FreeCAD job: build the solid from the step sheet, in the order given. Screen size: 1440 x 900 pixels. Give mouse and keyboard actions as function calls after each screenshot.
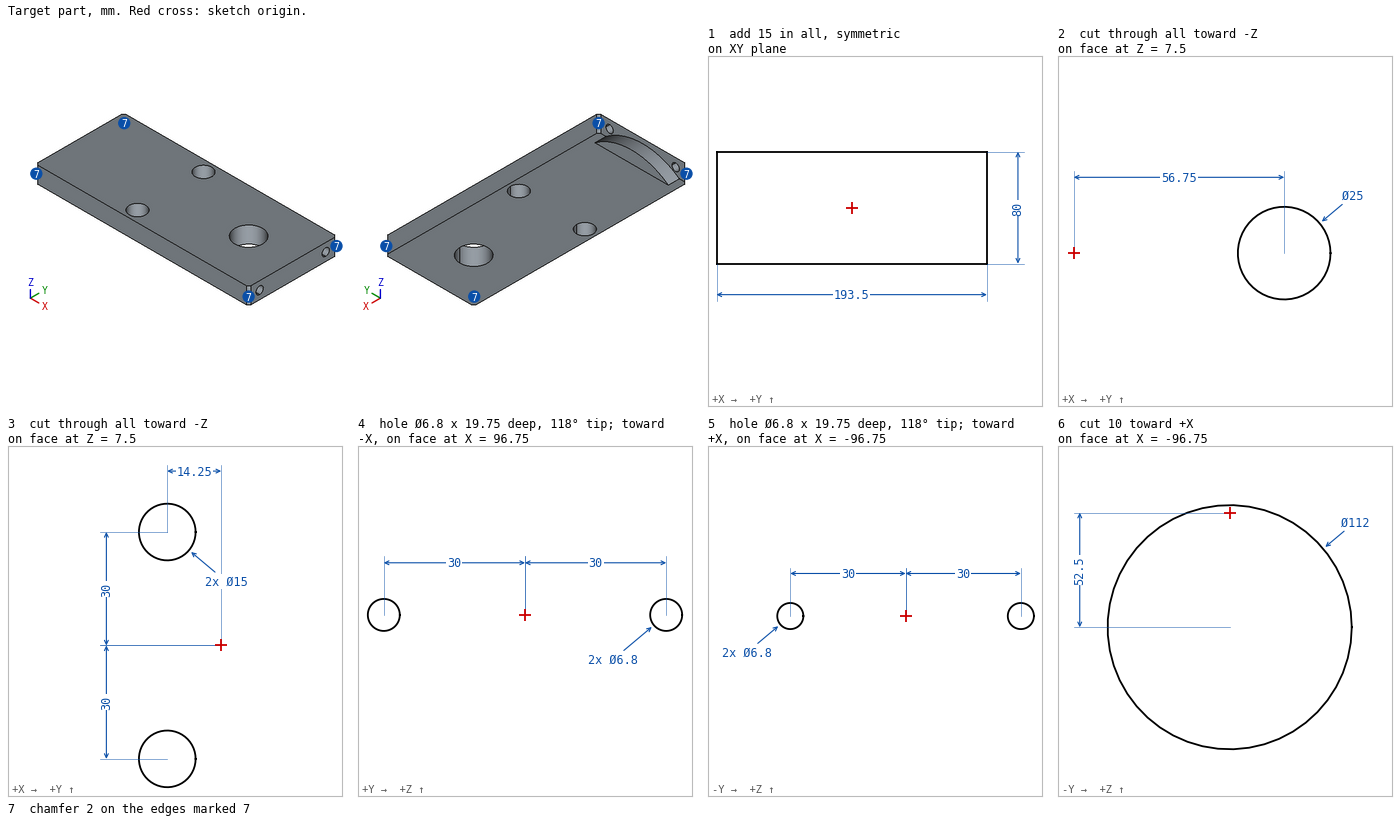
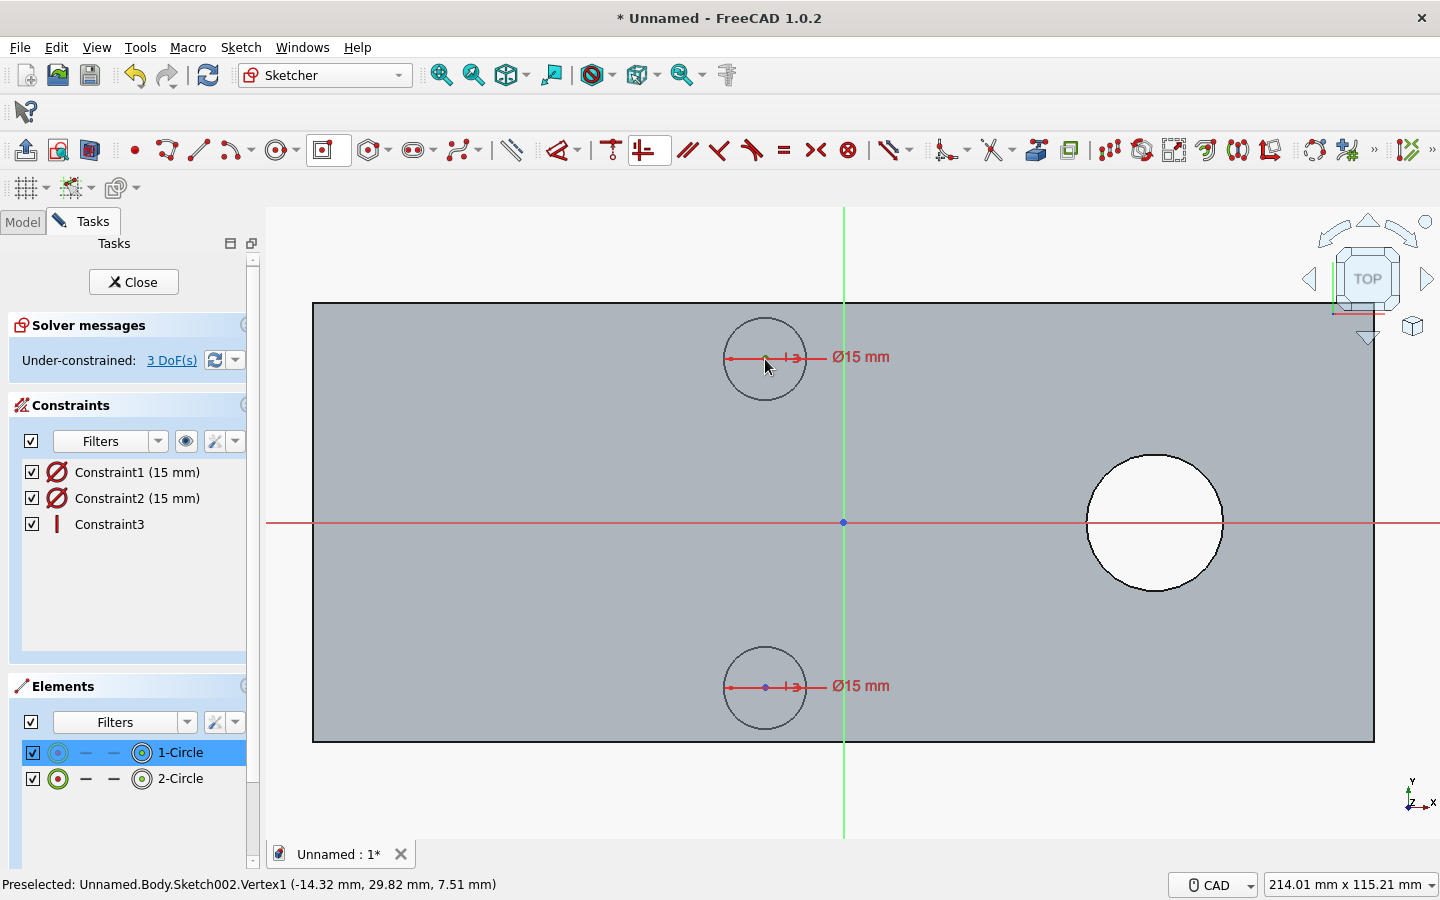
click(580, 150)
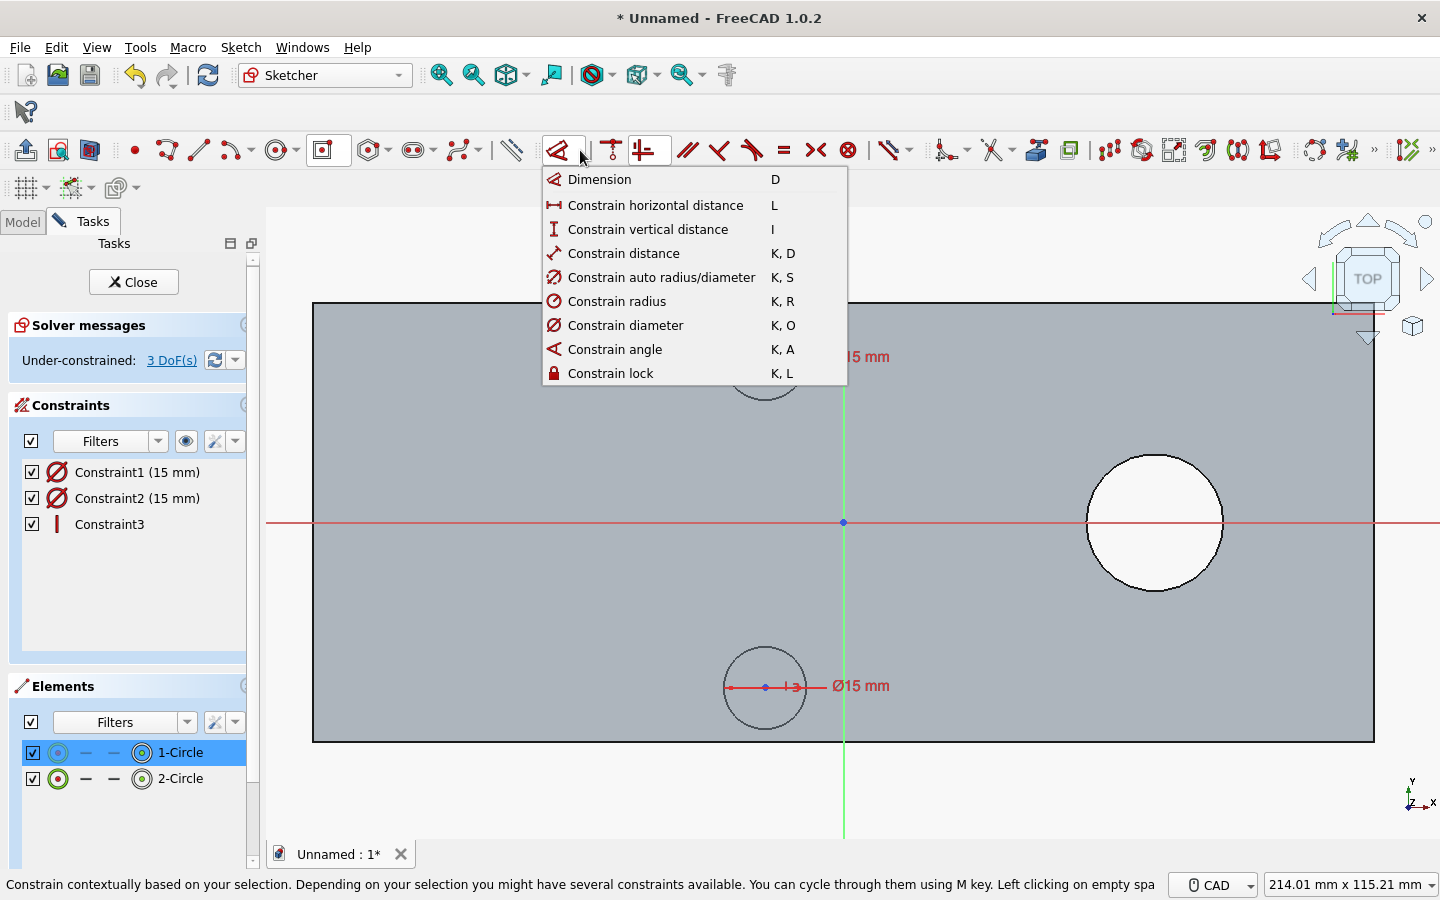
click(695, 229)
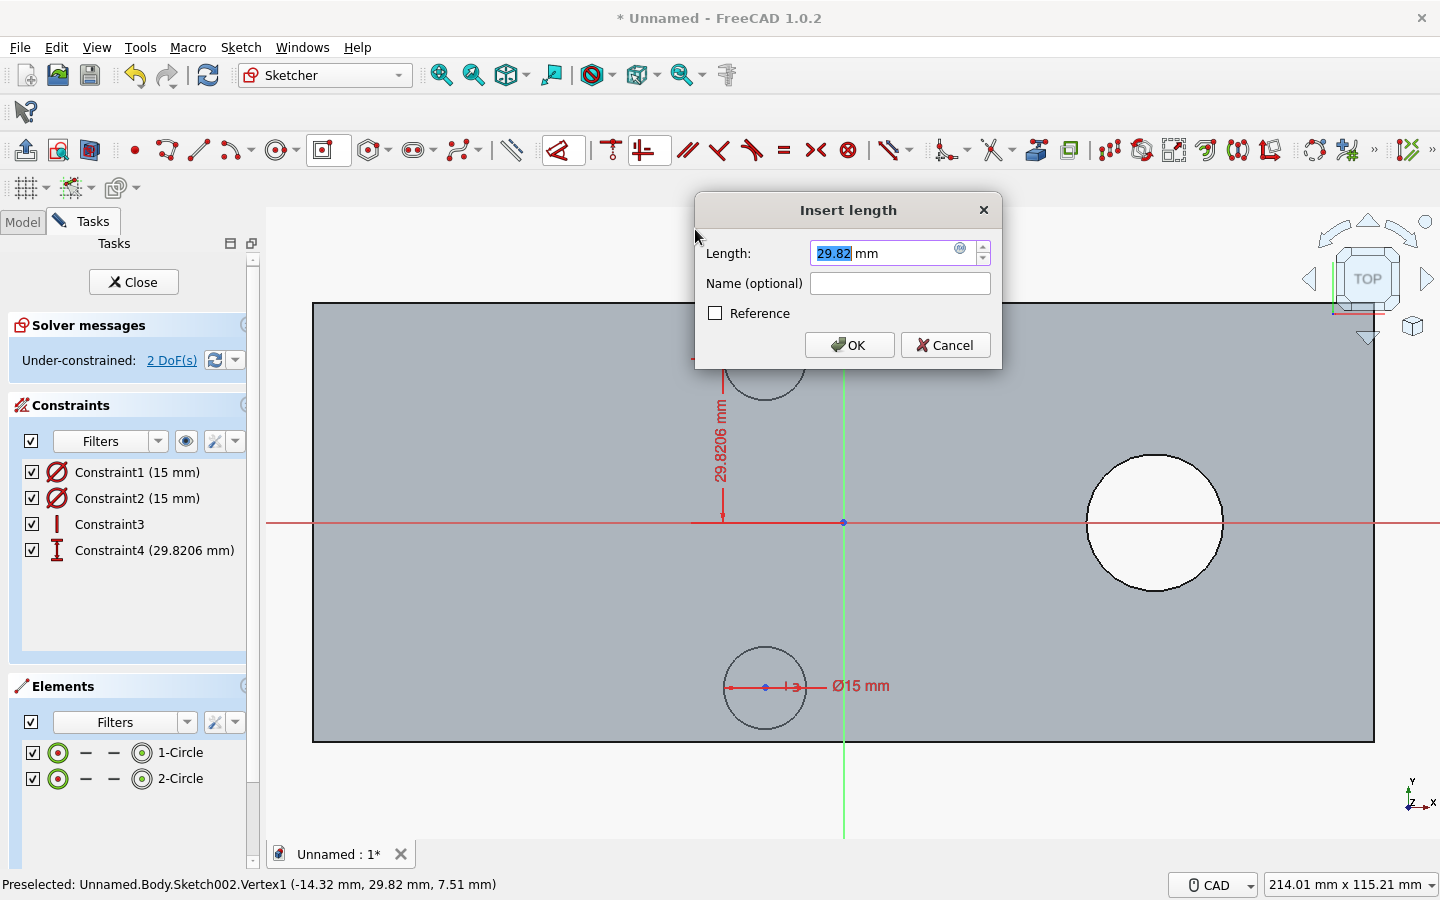
text(30)
key(Return)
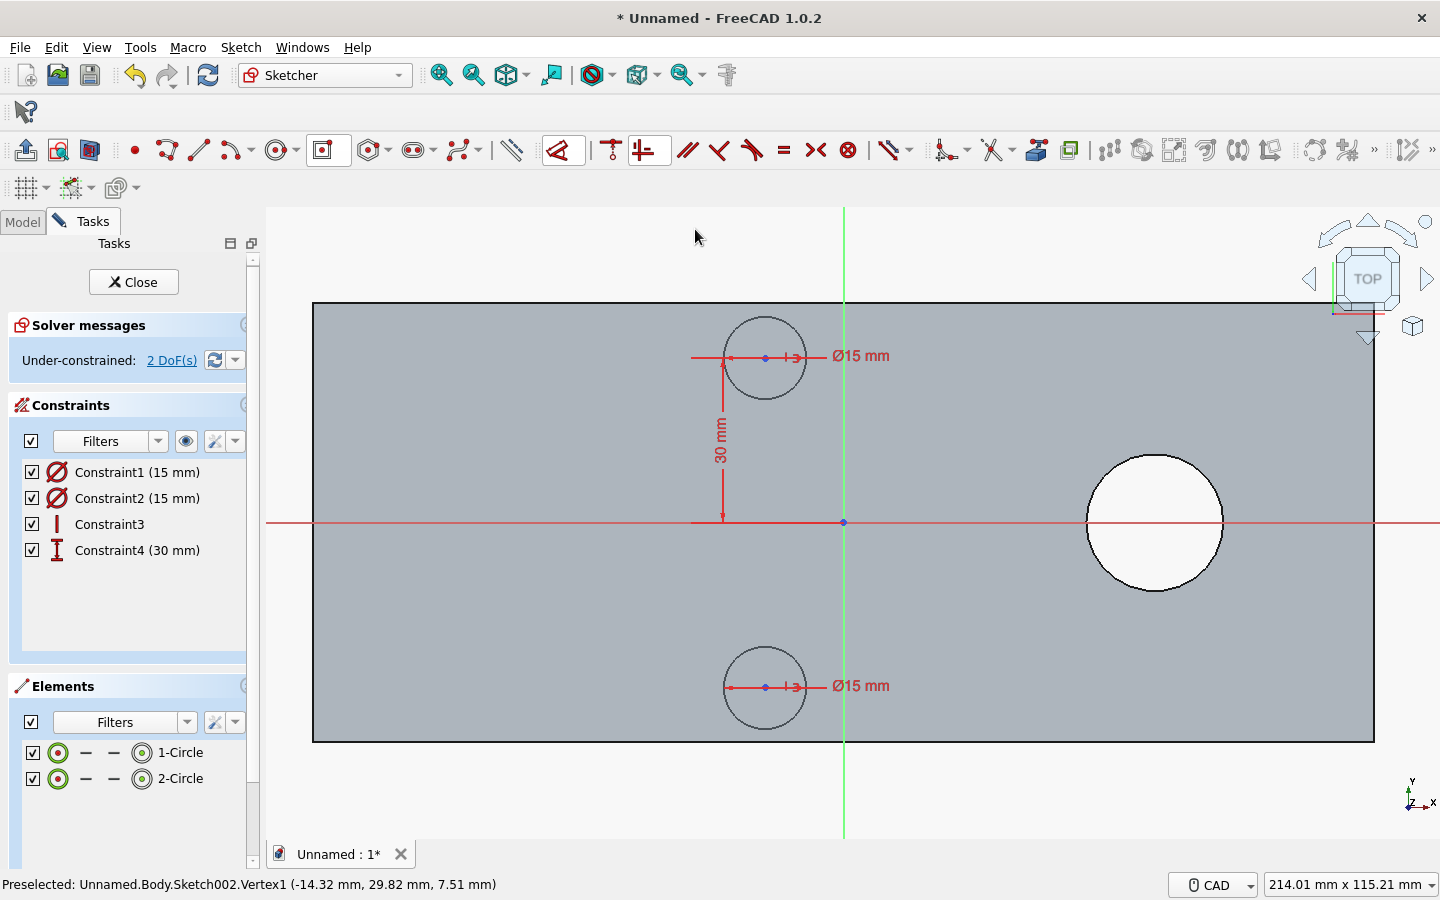
click(765, 688)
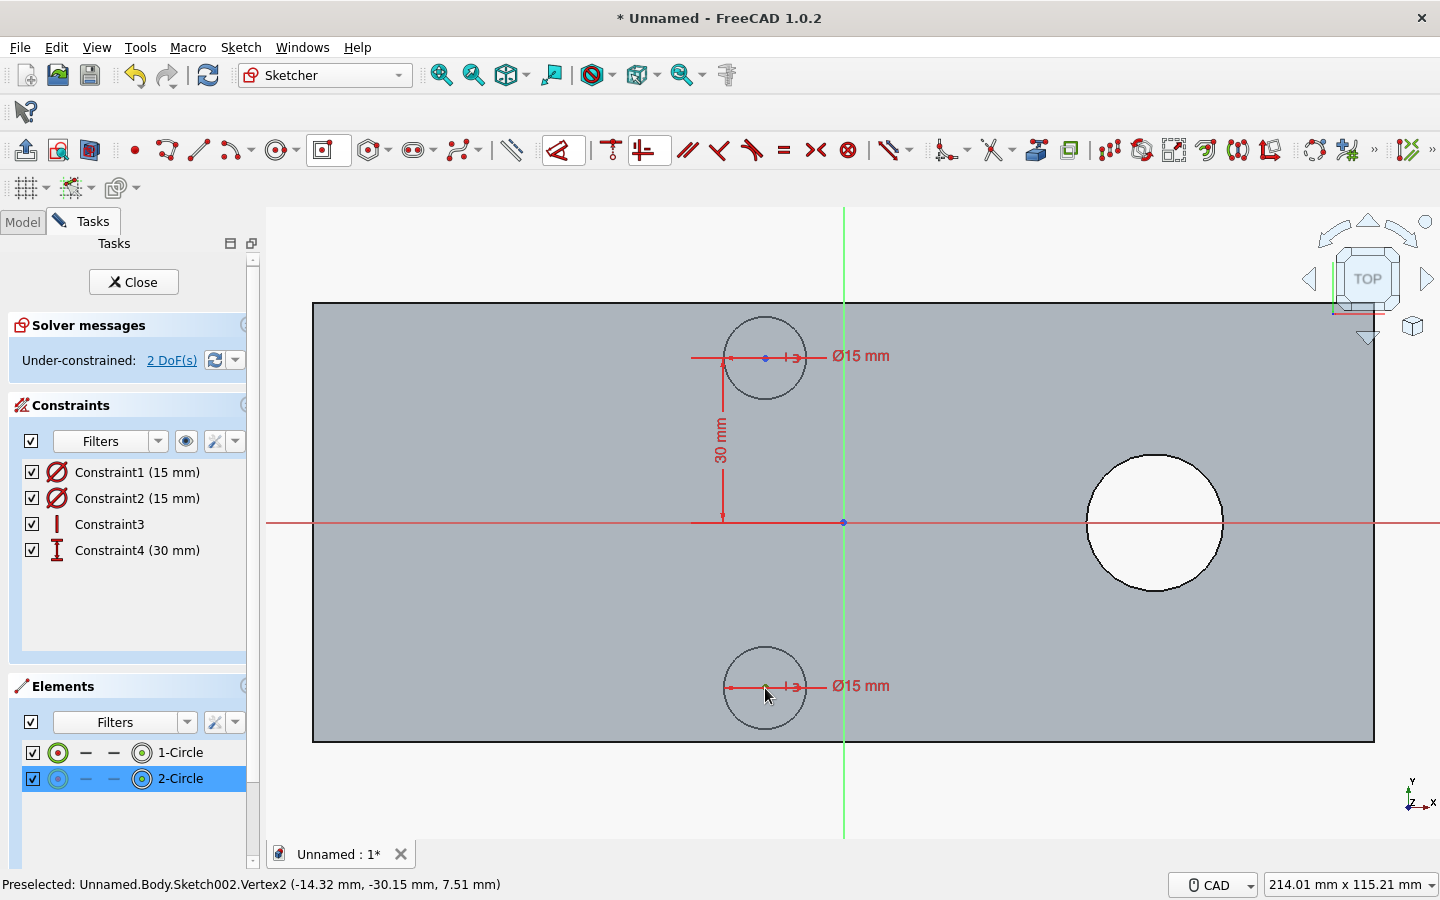
click(580, 150)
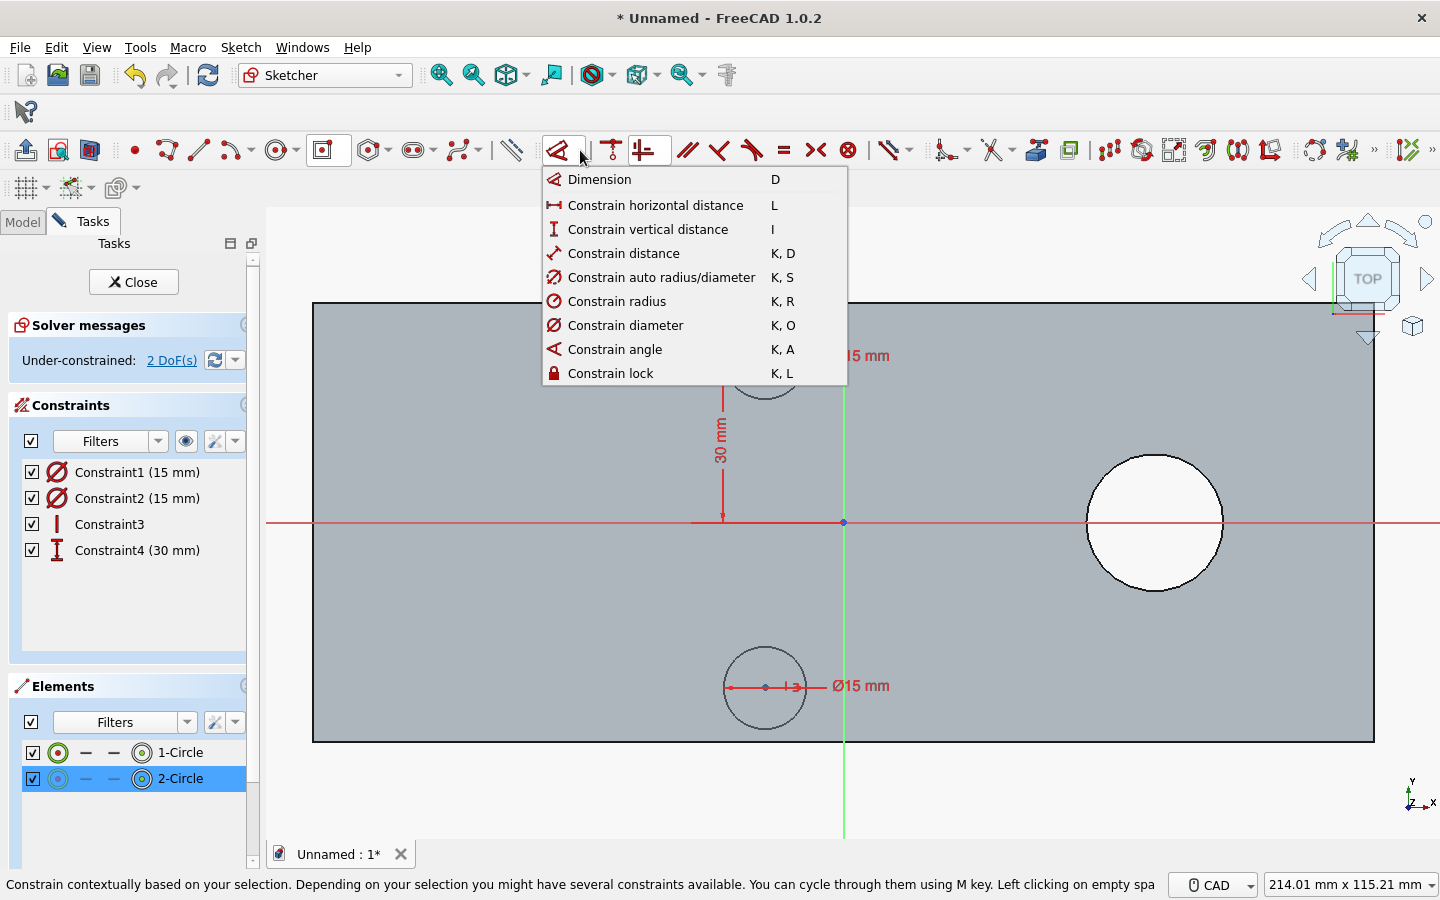
click(695, 229)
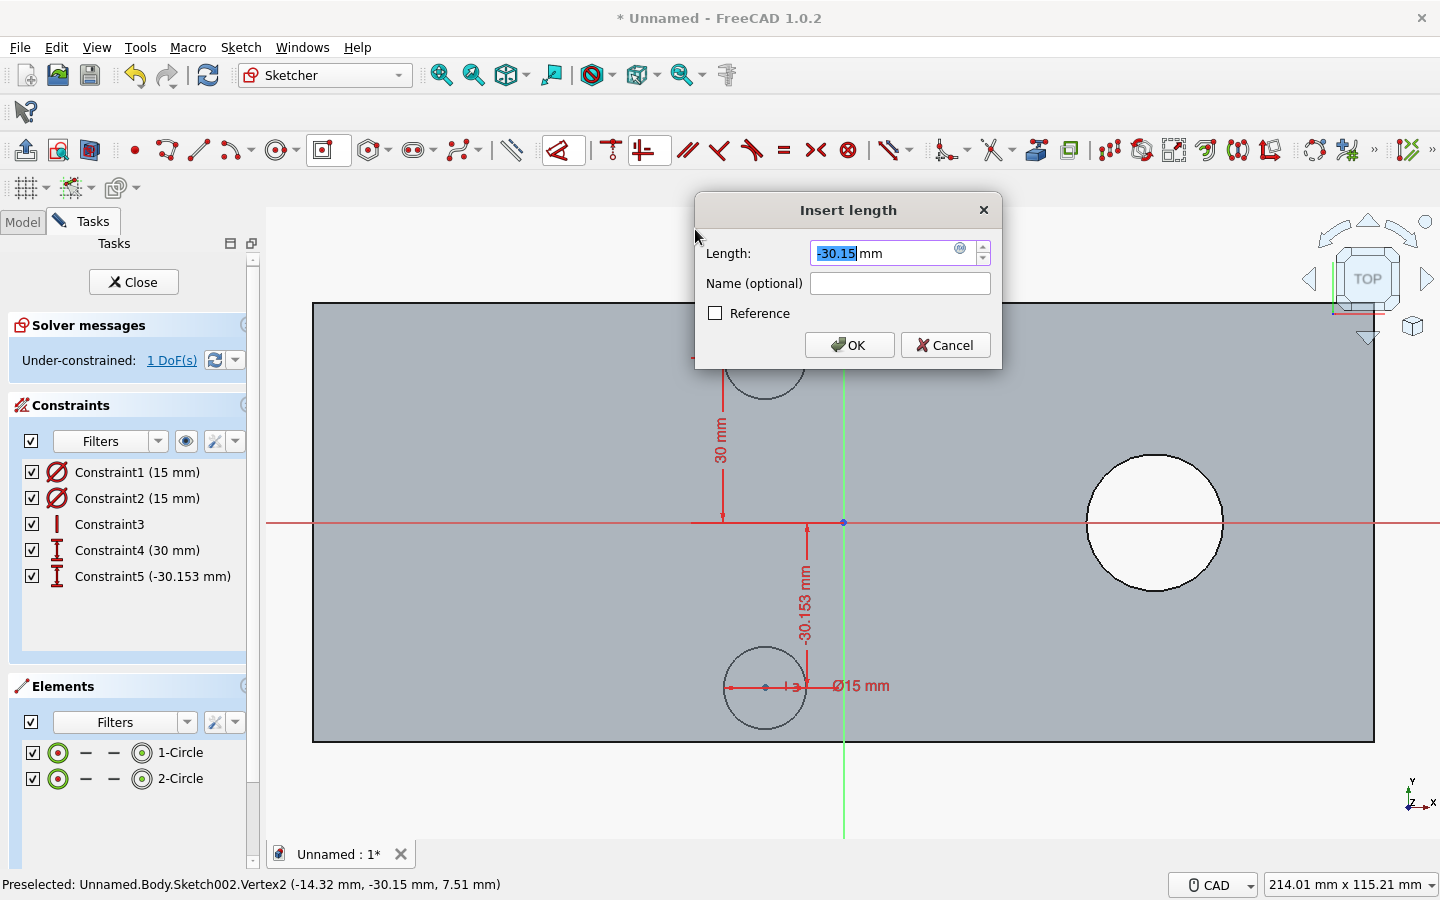
text(-30)
key(Return)